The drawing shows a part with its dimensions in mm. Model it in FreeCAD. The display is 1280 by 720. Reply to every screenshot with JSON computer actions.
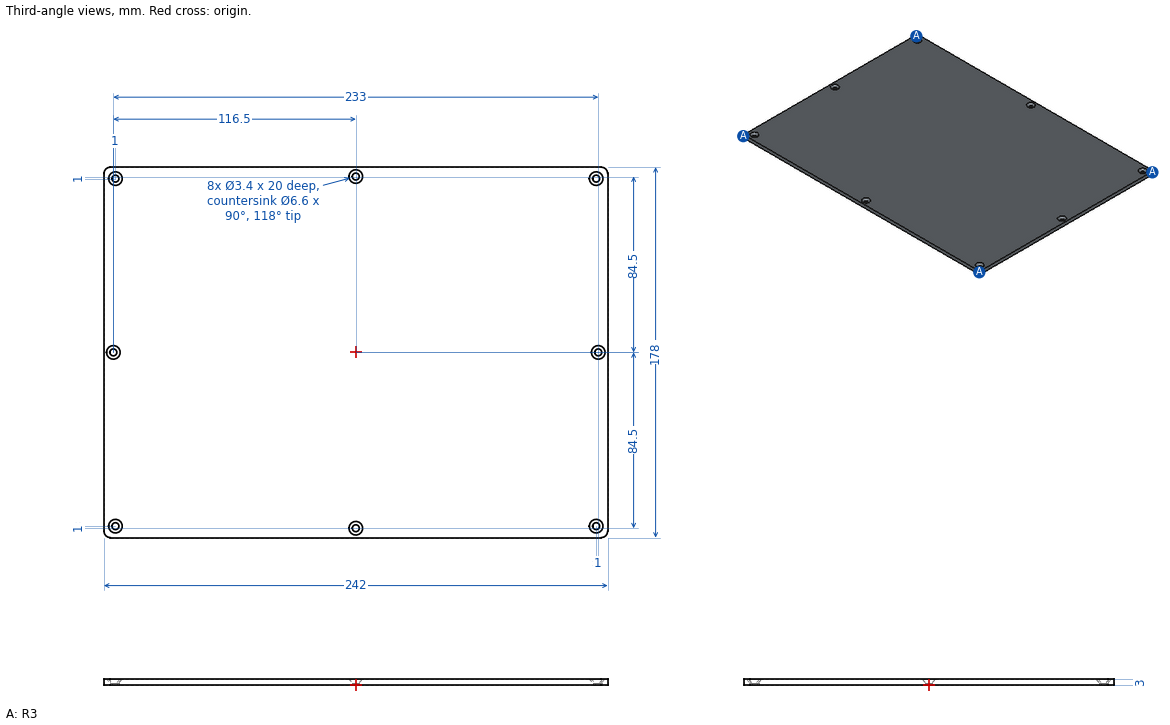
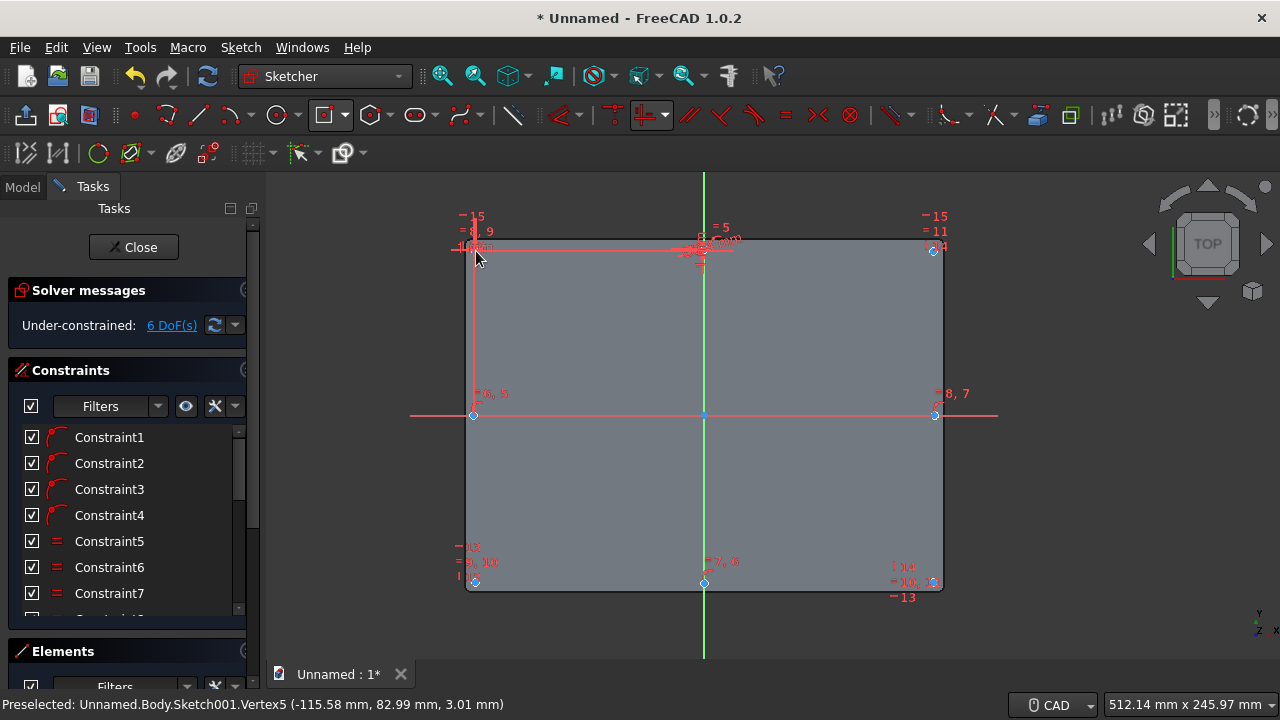
{"action": "scroll", "coordinate": [704, 584], "scroll_direction": "up", "scroll_amount": 15}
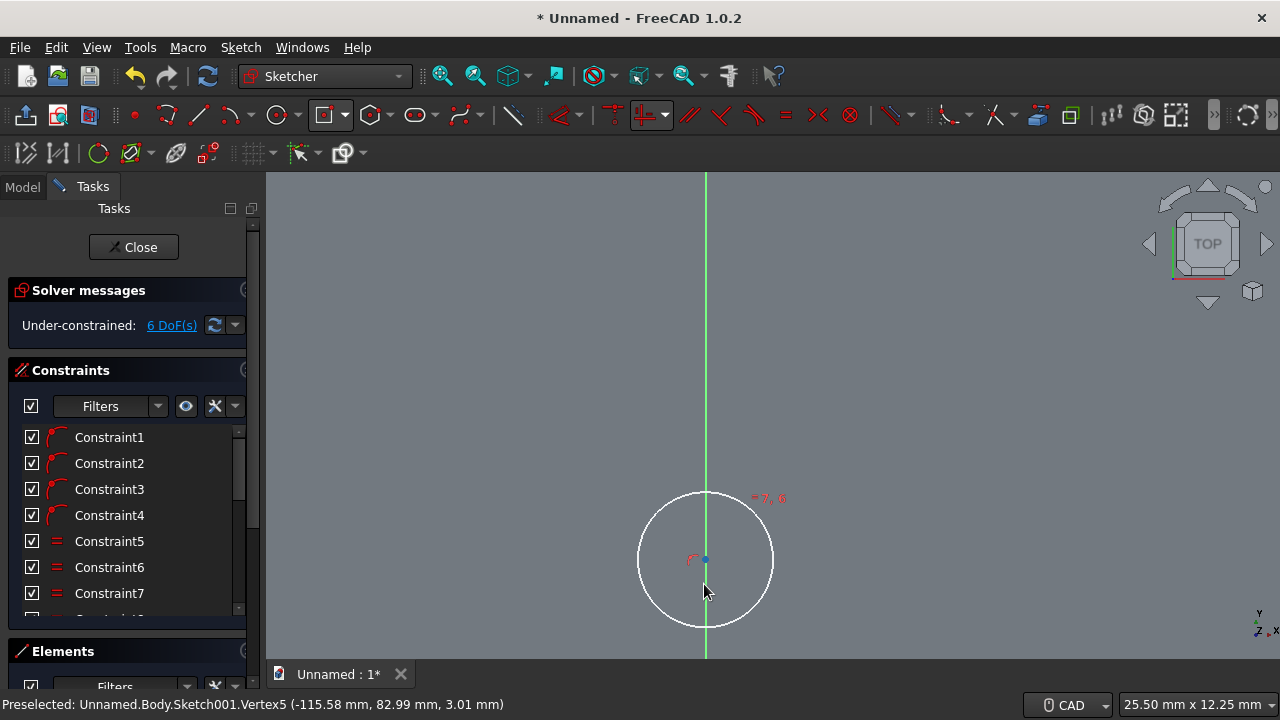
{"action": "left_click", "coordinate": [706, 560]}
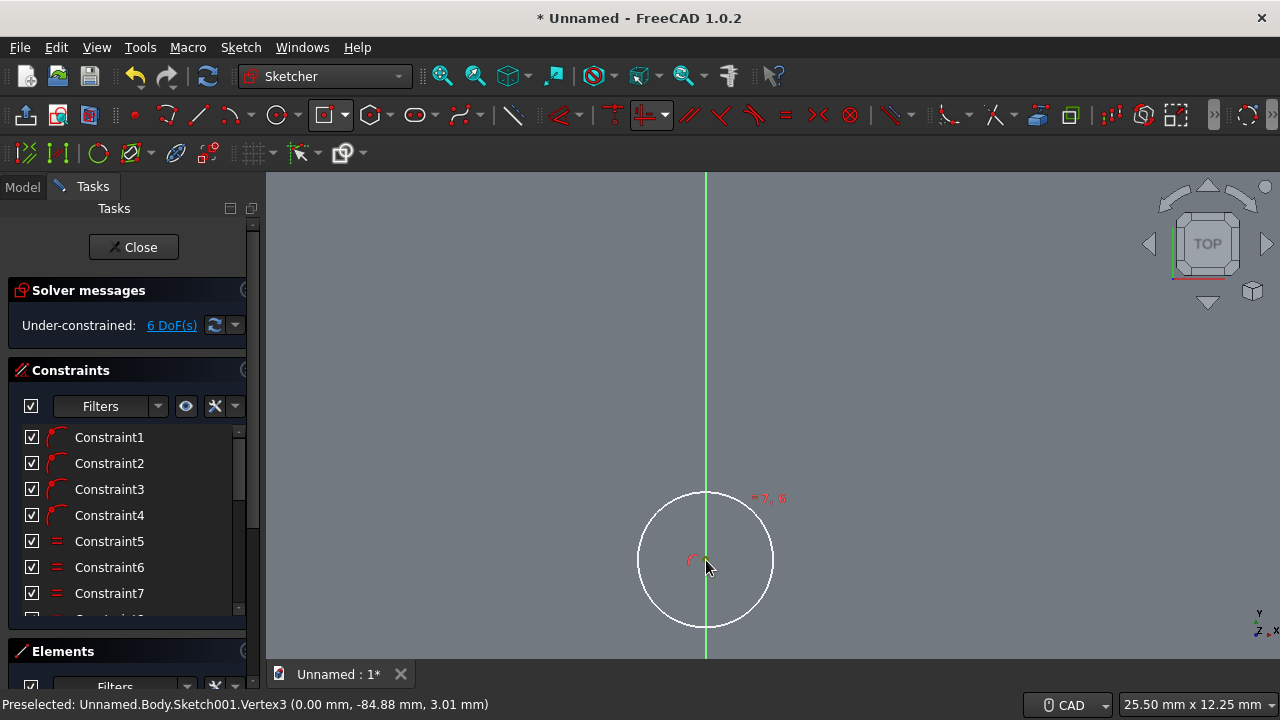
{"action": "scroll", "coordinate": [704, 585], "scroll_direction": "down", "scroll_amount": 15}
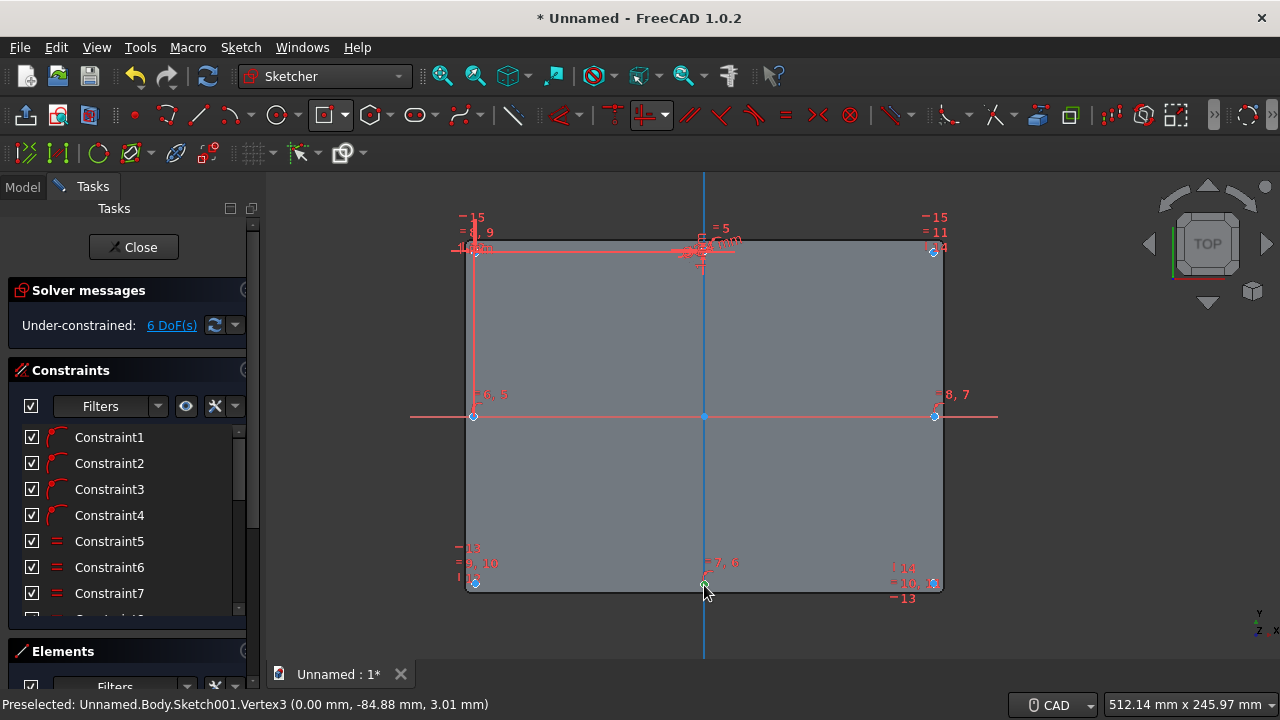
{"action": "scroll", "coordinate": [476, 583], "scroll_direction": "up", "scroll_amount": 15}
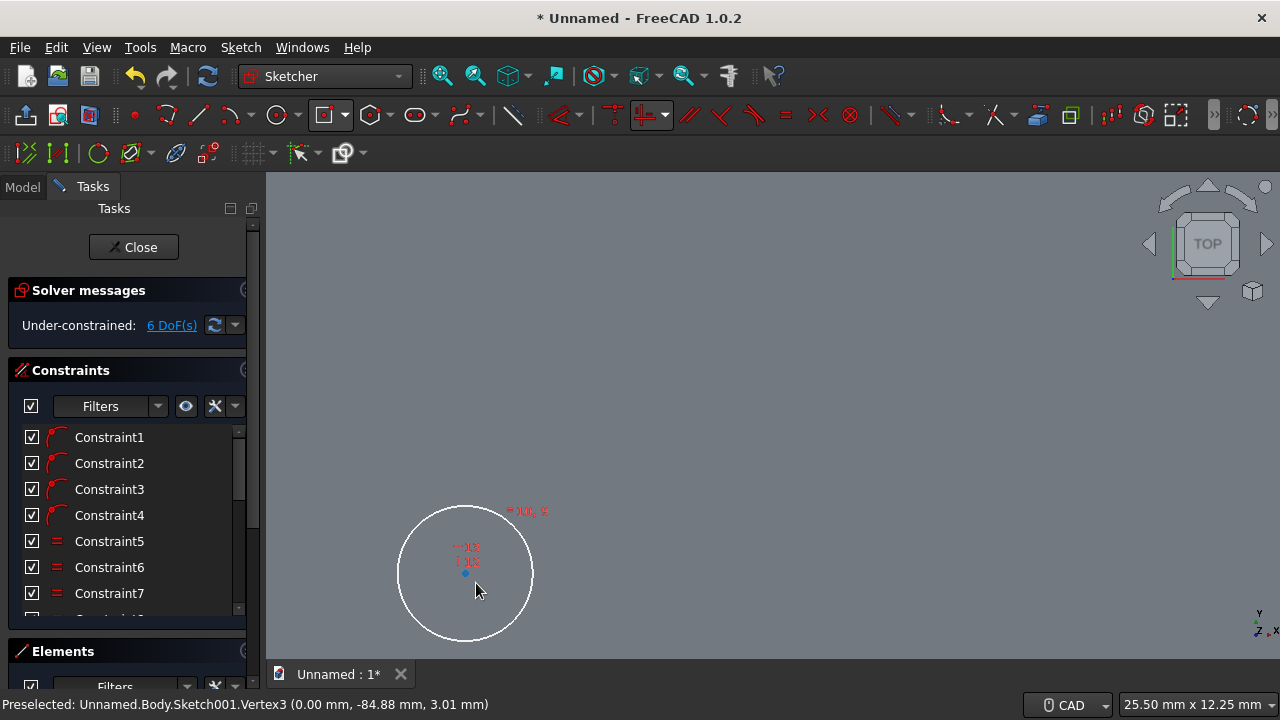
{"action": "left_click", "coordinate": [465, 574]}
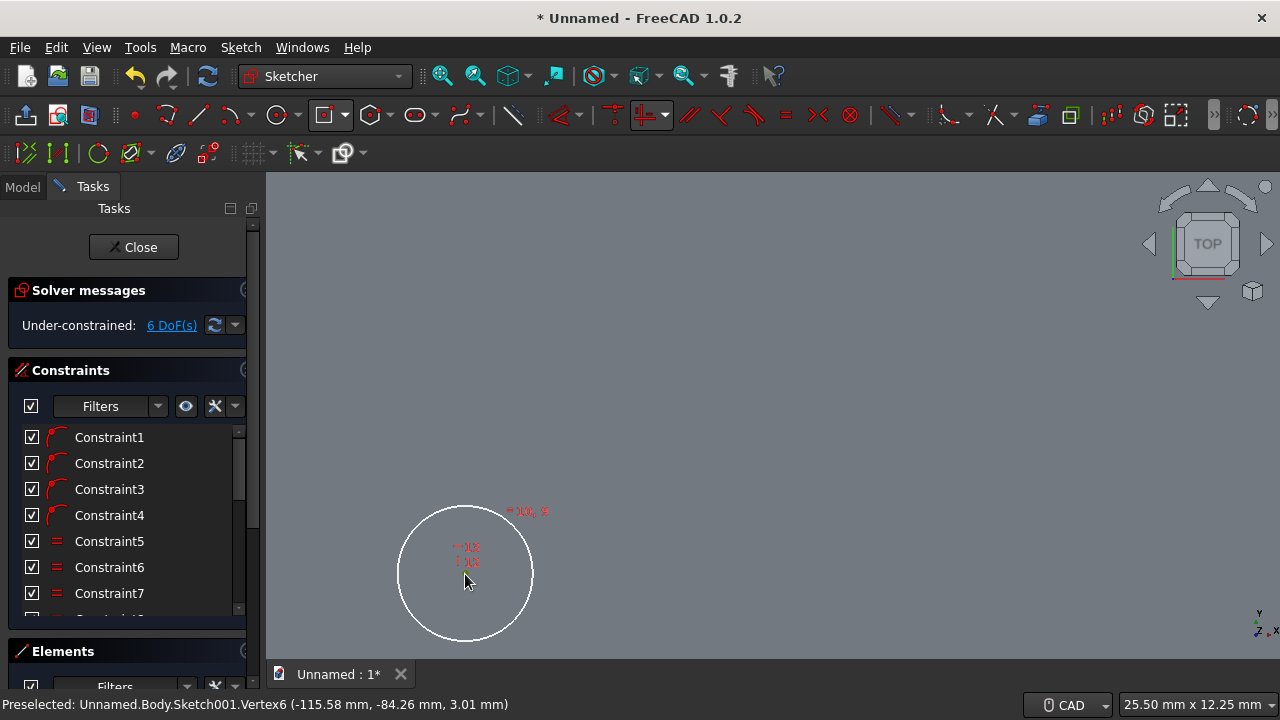
{"action": "key", "text": "i"}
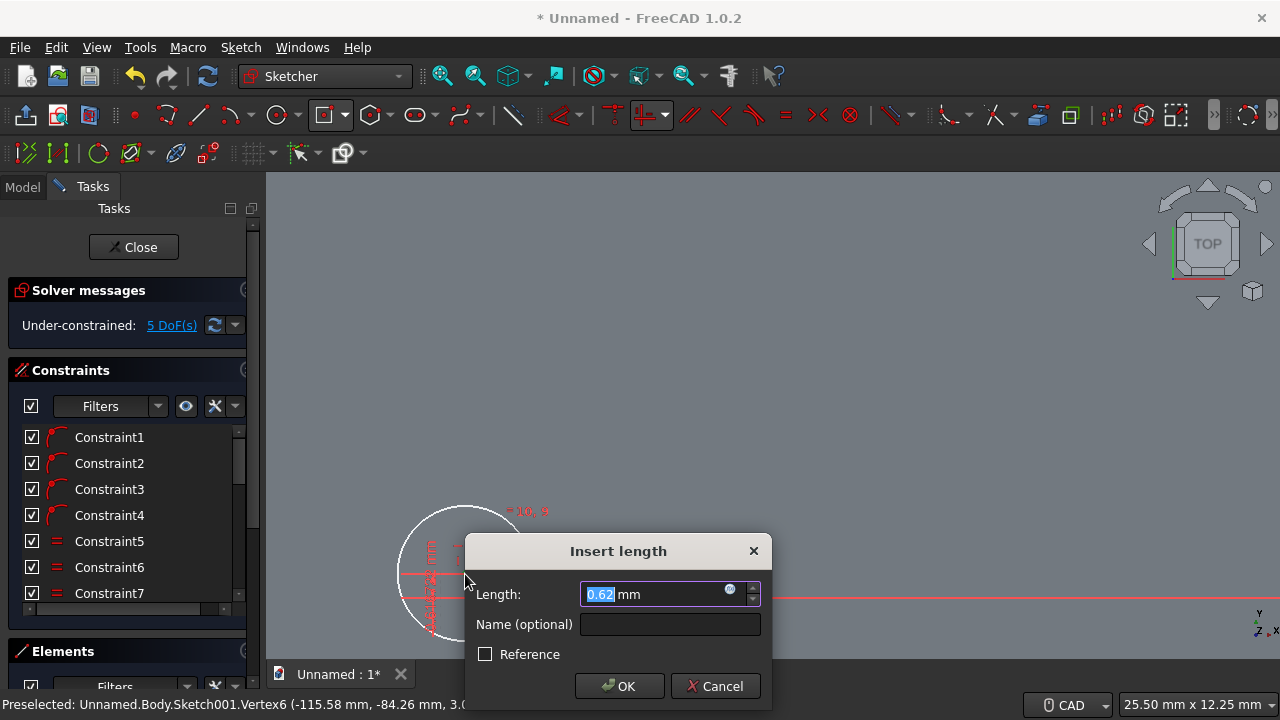
{"action": "type", "text": "1"}
{"action": "key", "text": "Return"}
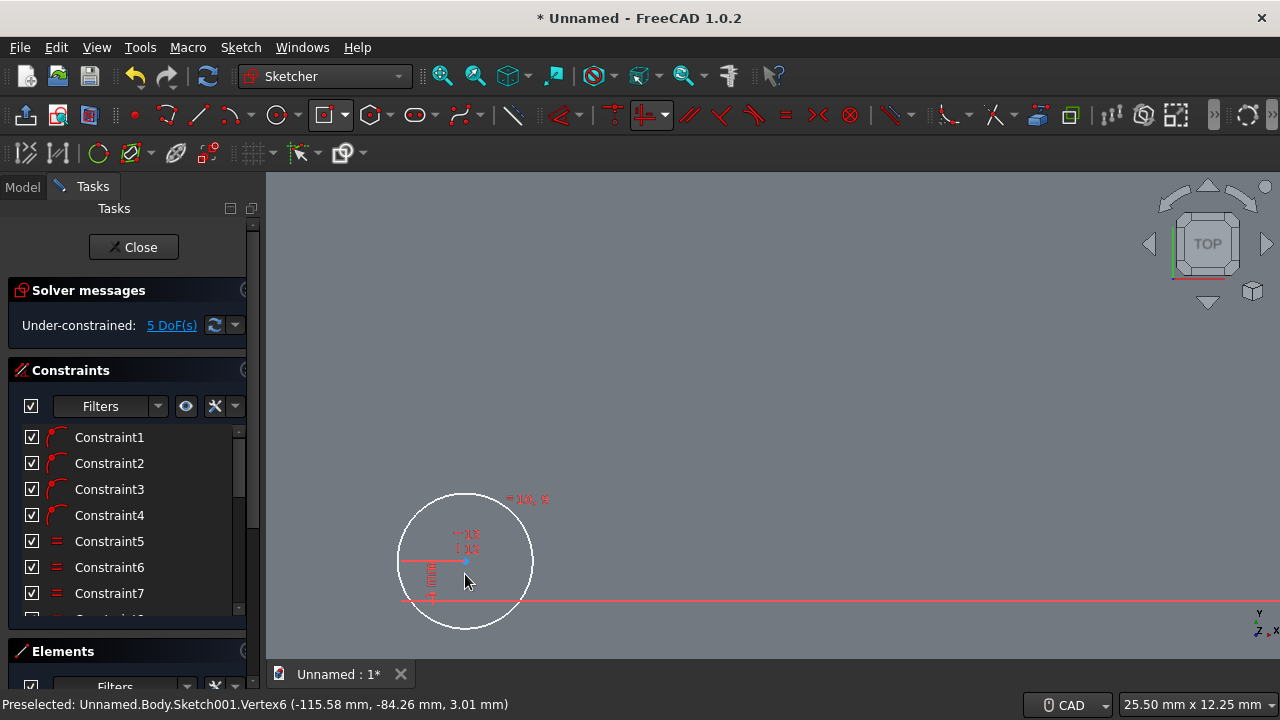
{"action": "scroll", "coordinate": [476, 583], "scroll_direction": "down", "scroll_amount": 15}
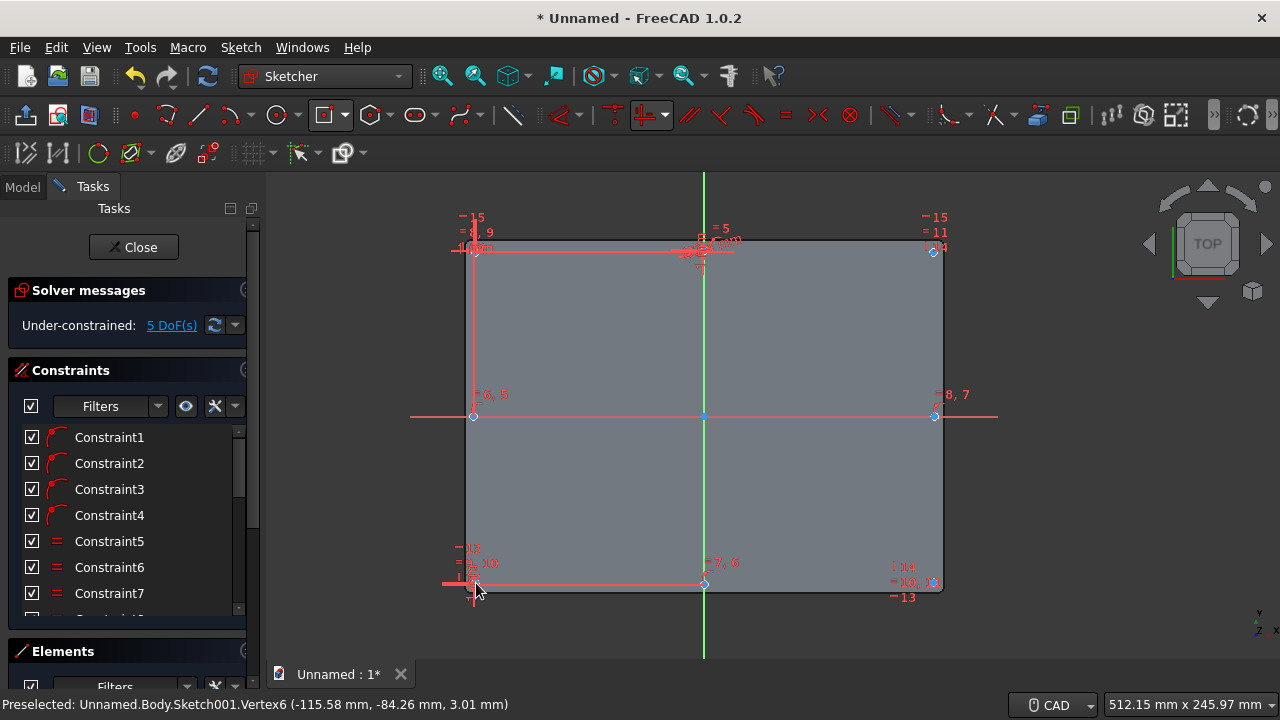
{"action": "scroll", "coordinate": [935, 417], "scroll_direction": "up", "scroll_amount": 15}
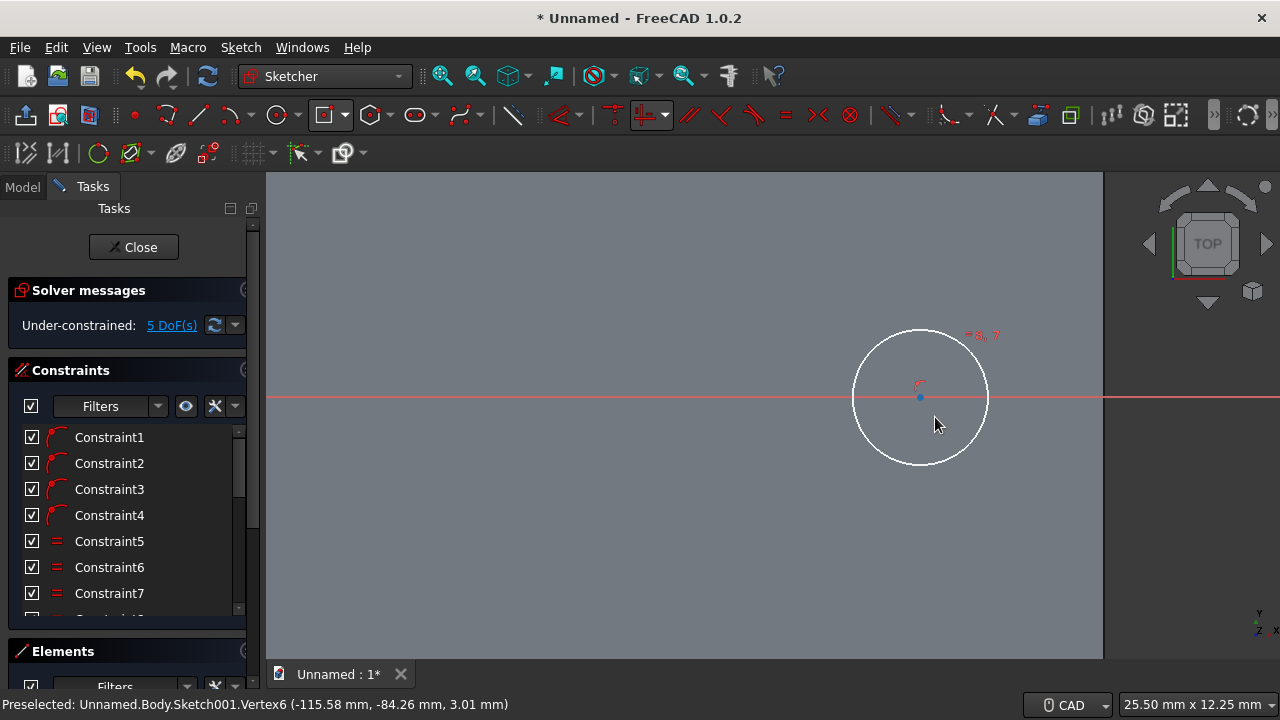
{"action": "left_click", "coordinate": [920, 397]}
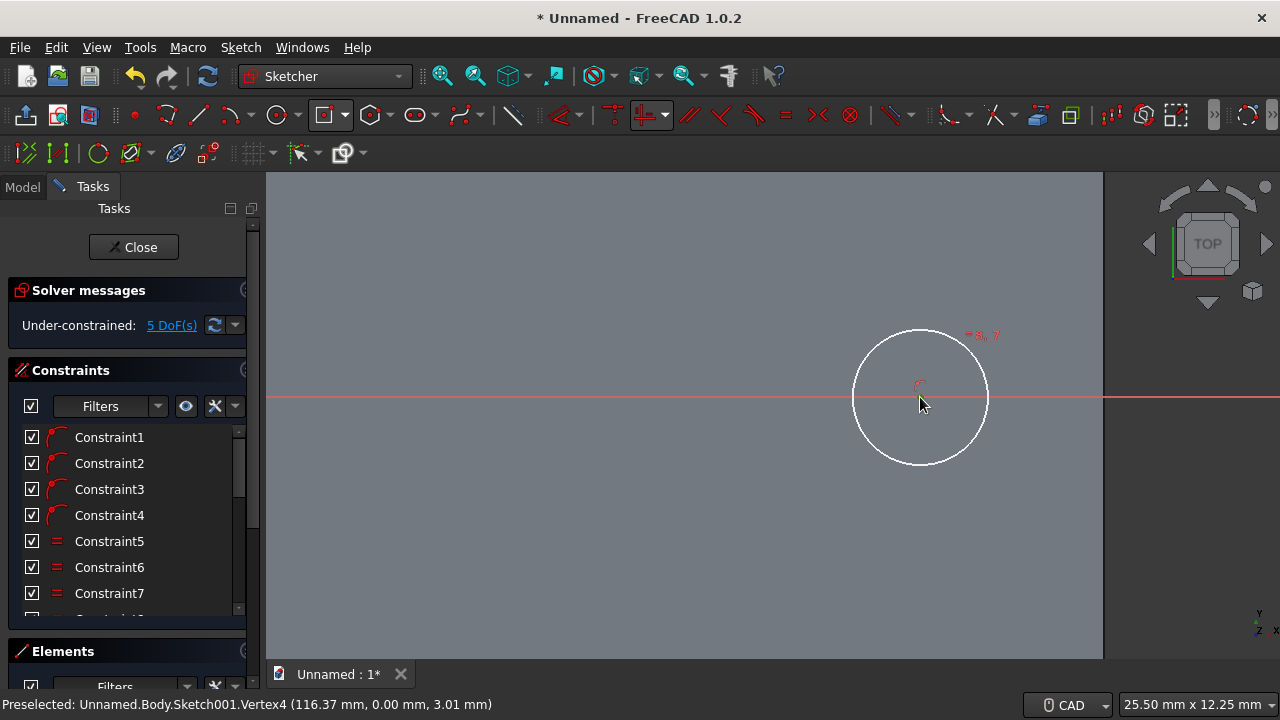
{"action": "scroll", "coordinate": [936, 416], "scroll_direction": "down", "scroll_amount": 15}